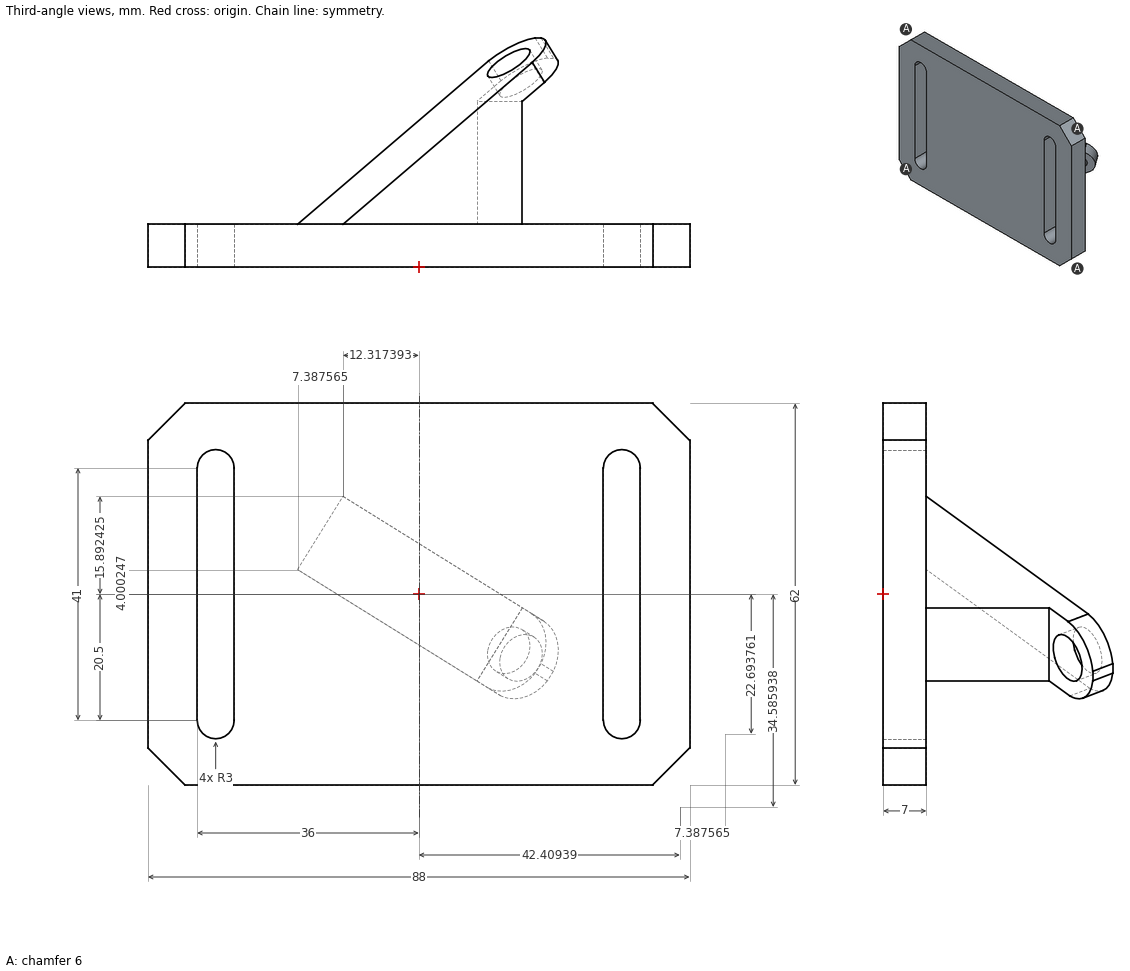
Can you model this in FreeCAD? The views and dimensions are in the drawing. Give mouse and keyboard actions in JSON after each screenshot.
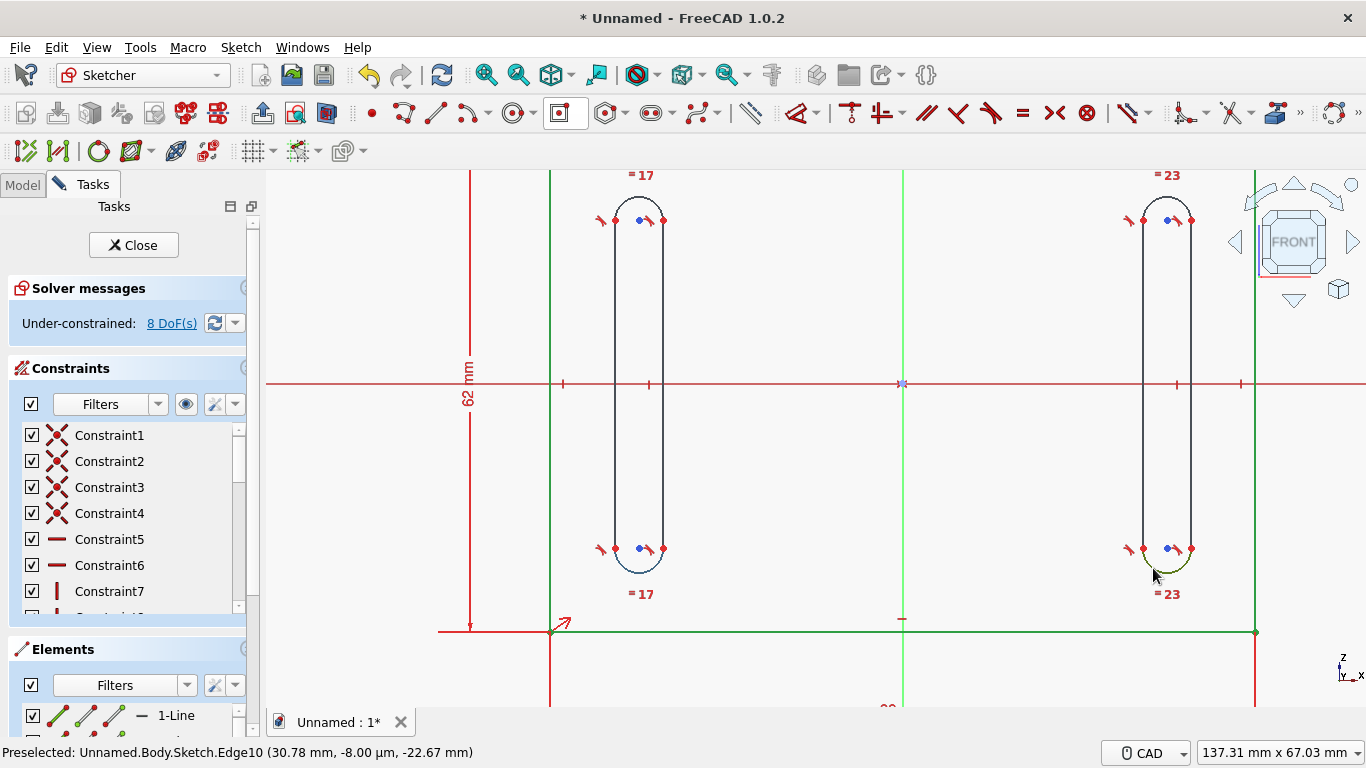
{"action": "left_click", "coordinate": [1024, 114]}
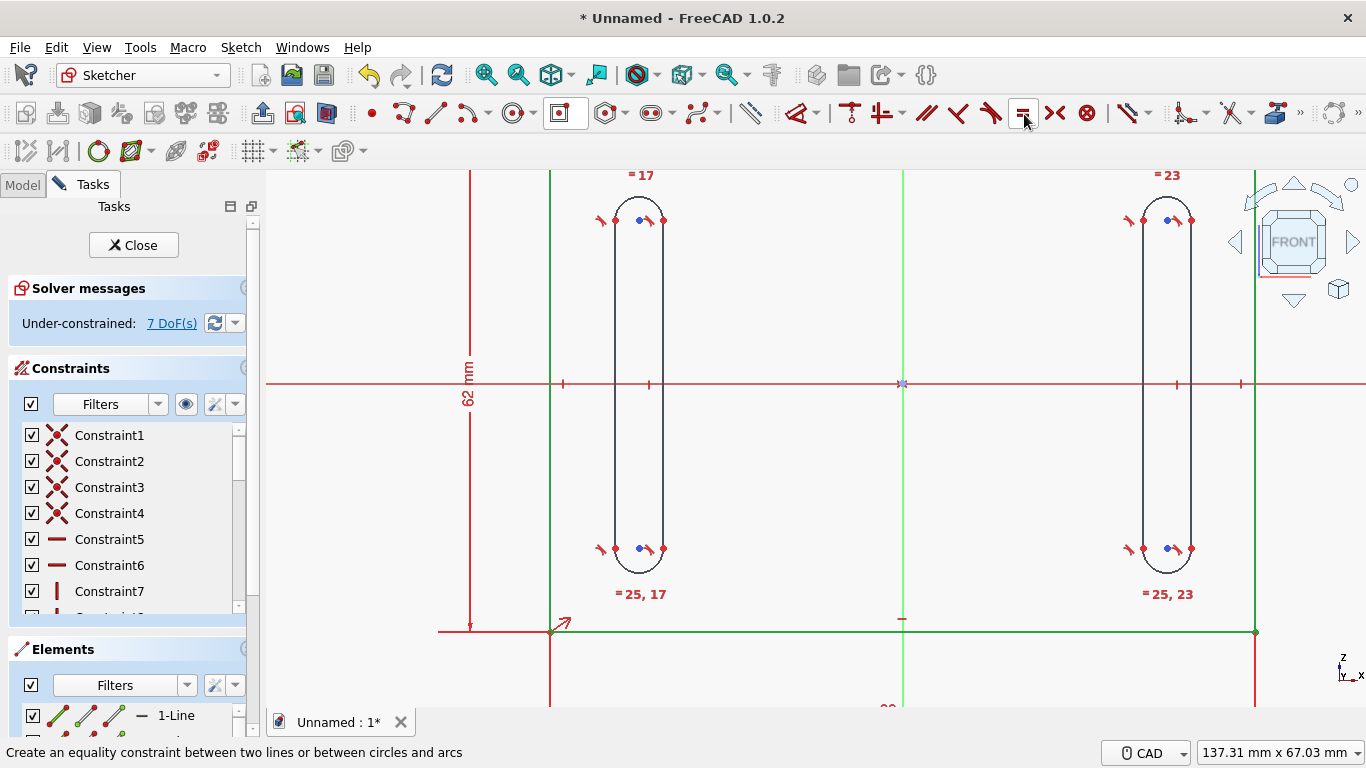
{"action": "left_click", "coordinate": [639, 549]}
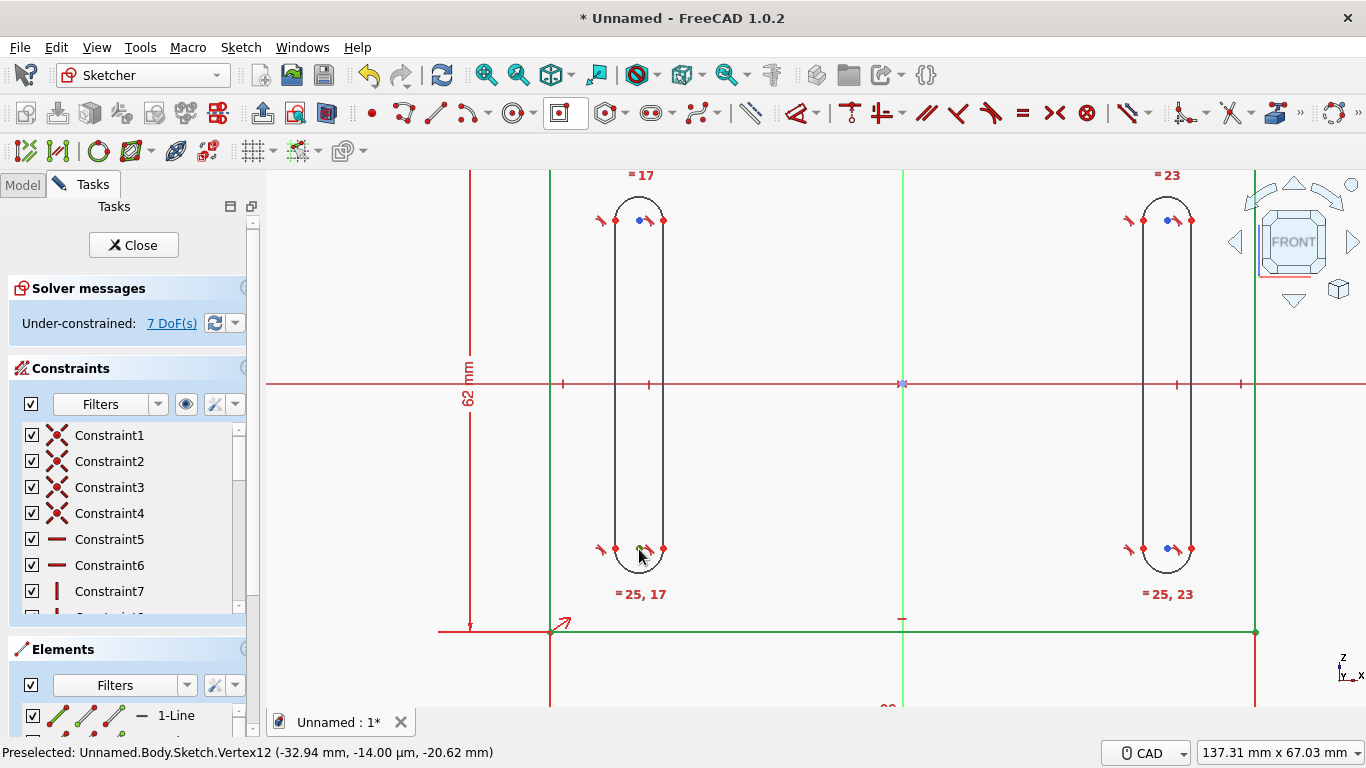
{"action": "left_click", "coordinate": [1167, 549]}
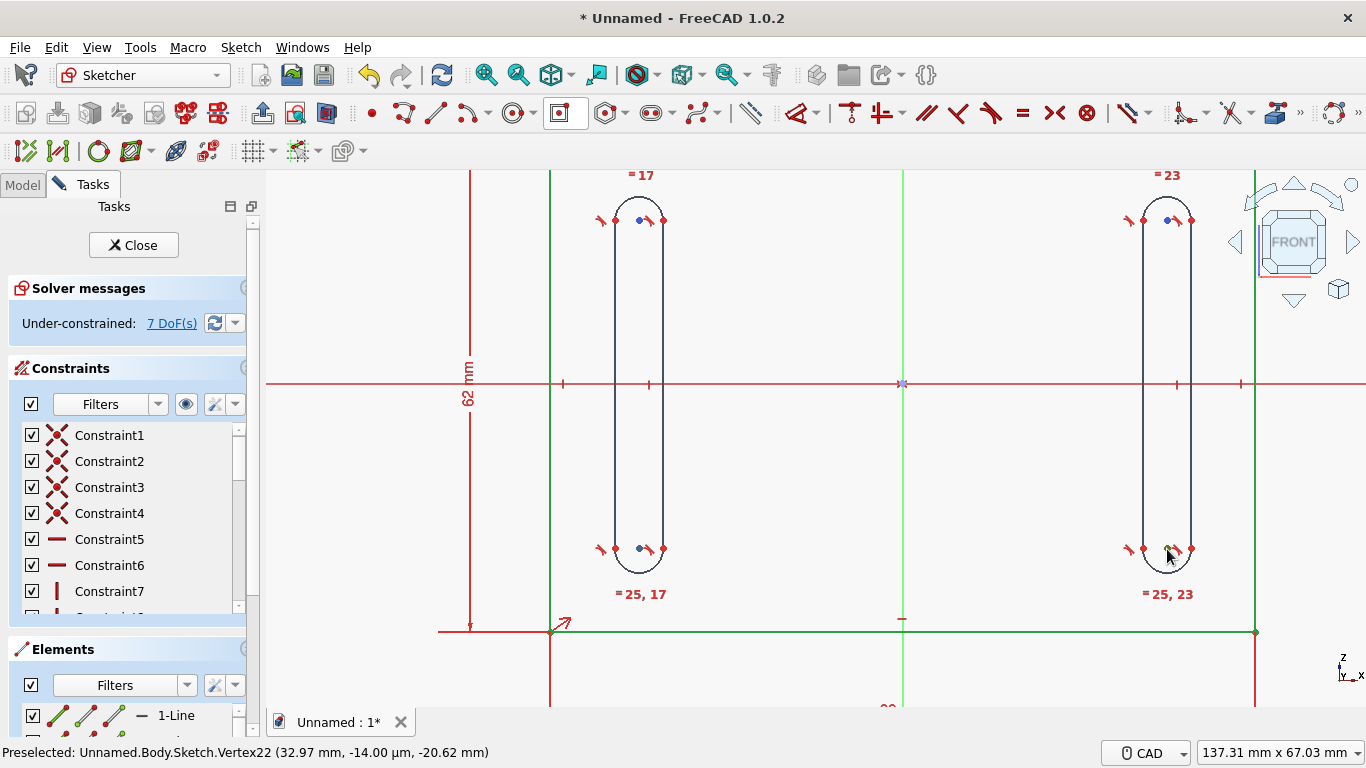
{"action": "left_click", "coordinate": [903, 576]}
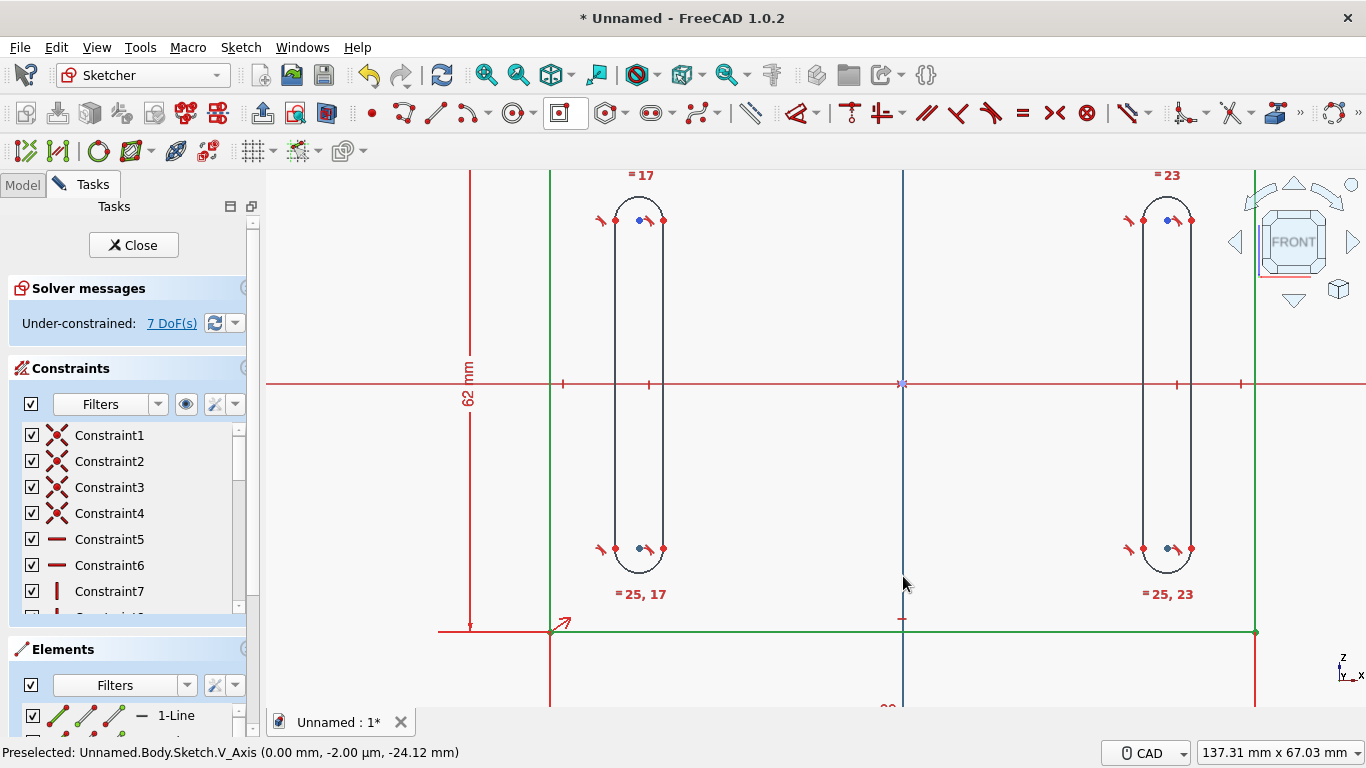
{"action": "left_click", "coordinate": [1056, 114]}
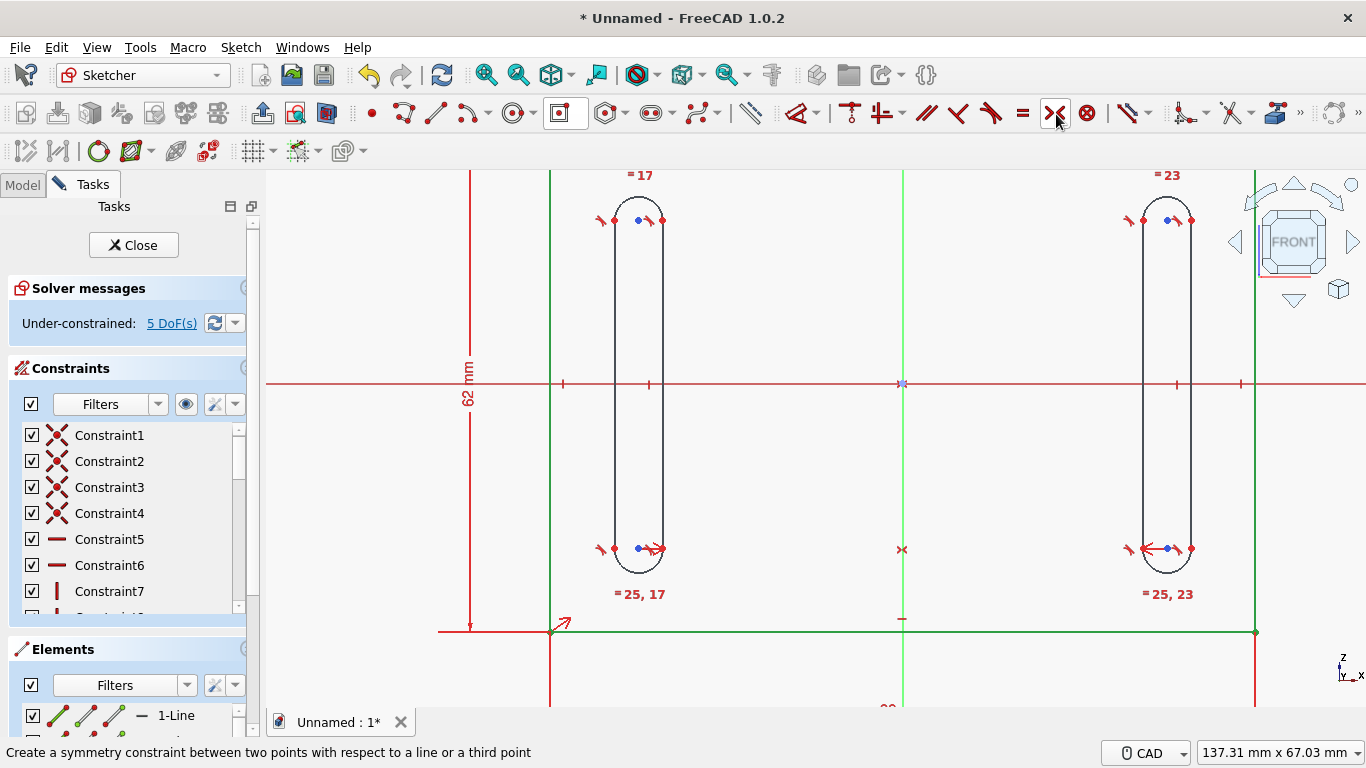
{"action": "left_click", "coordinate": [796, 114]}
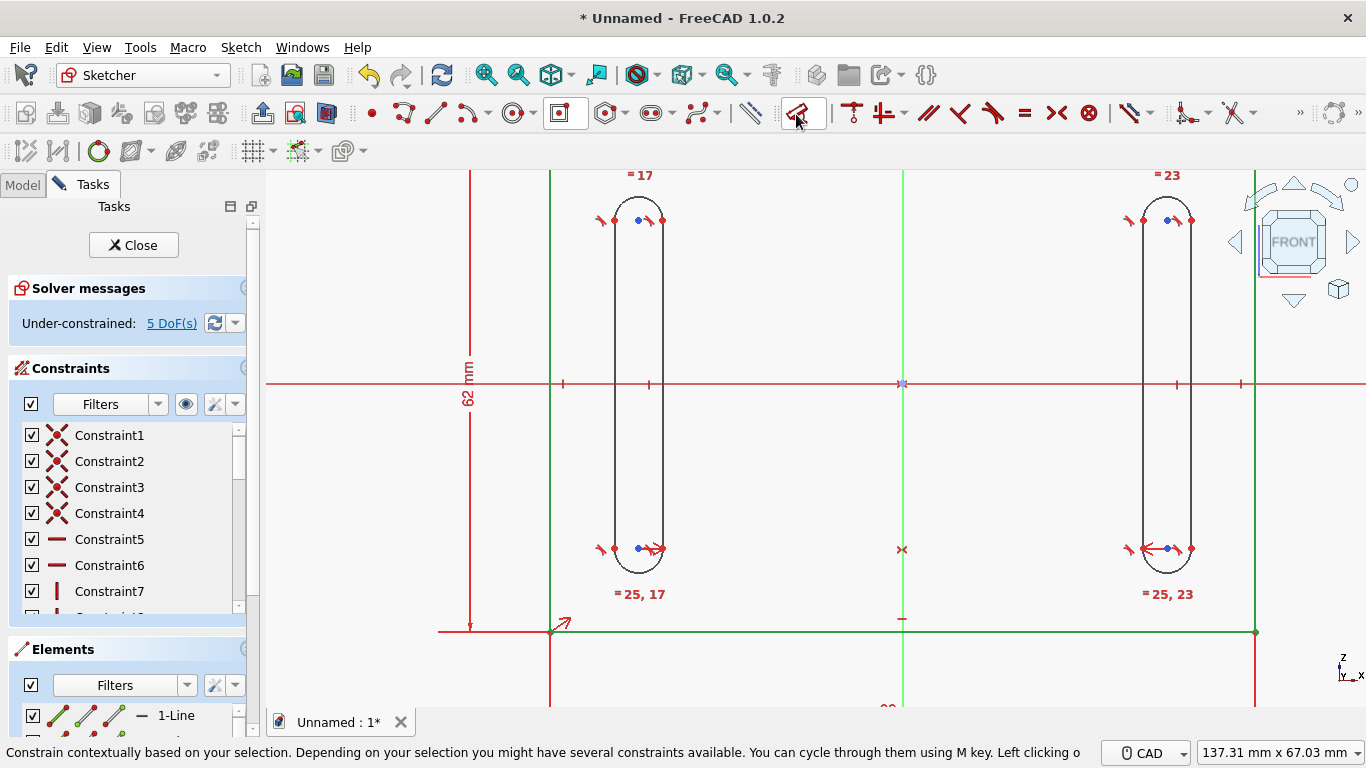
{"action": "scroll", "coordinate": [625, 568], "scroll_direction": "up", "scroll_amount": 3}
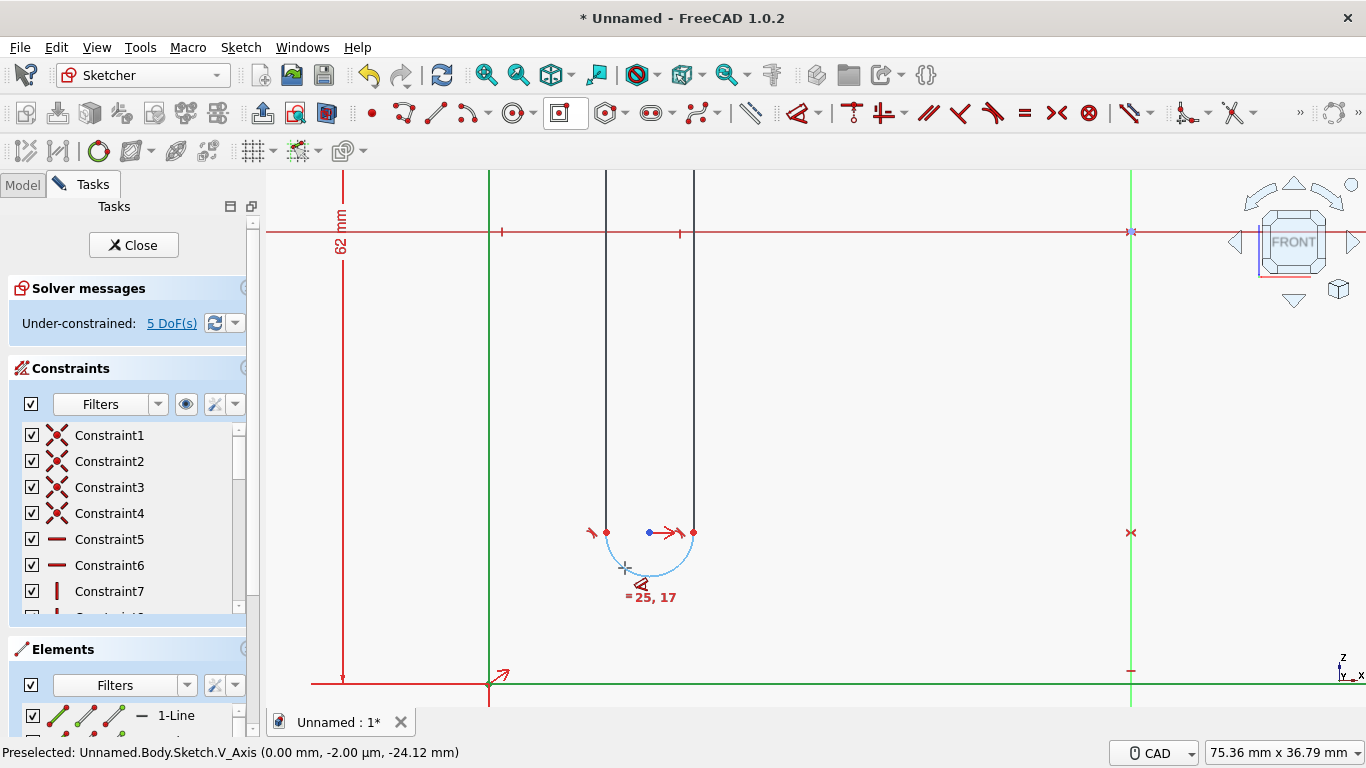
{"action": "left_click", "coordinate": [624, 568]}
{"action": "left_click", "coordinate": [605, 594]}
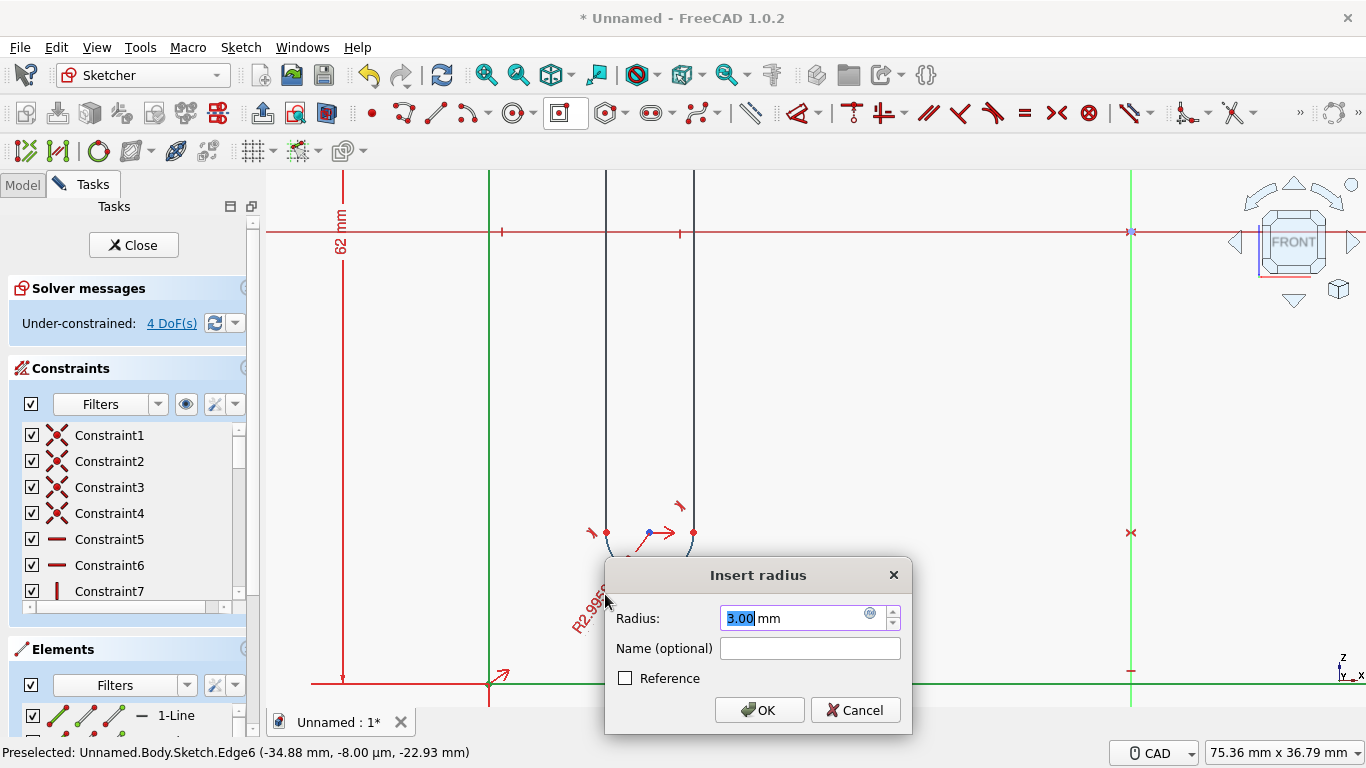
{"action": "type", "text": "3"}
{"action": "key", "text": "Return"}